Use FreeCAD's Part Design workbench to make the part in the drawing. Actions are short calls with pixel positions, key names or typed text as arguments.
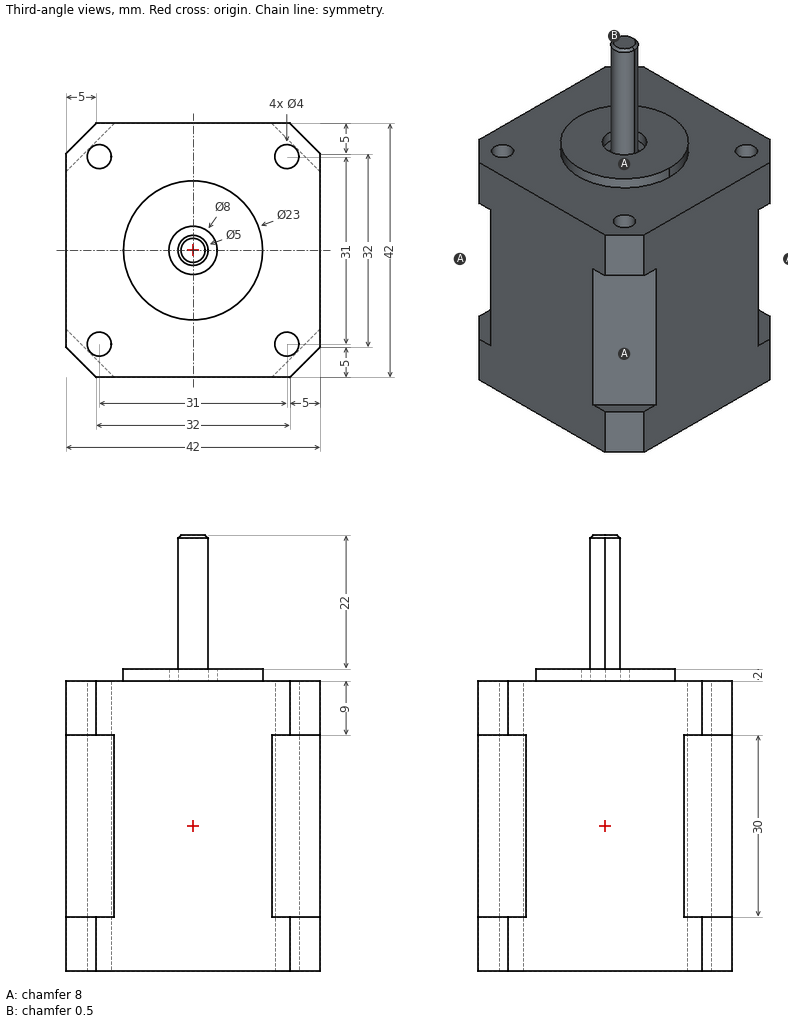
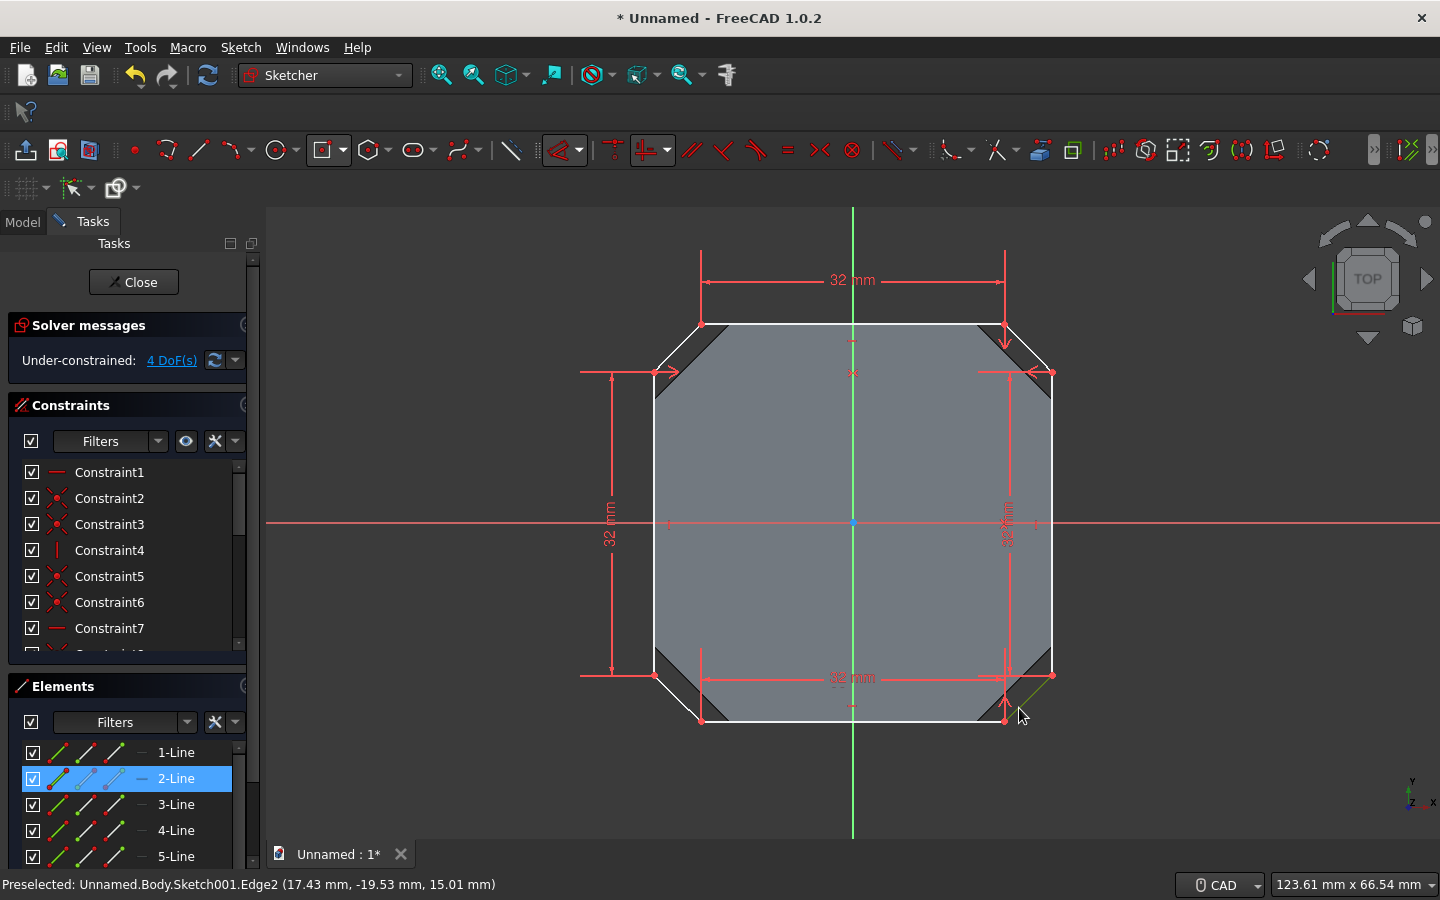
click(582, 150)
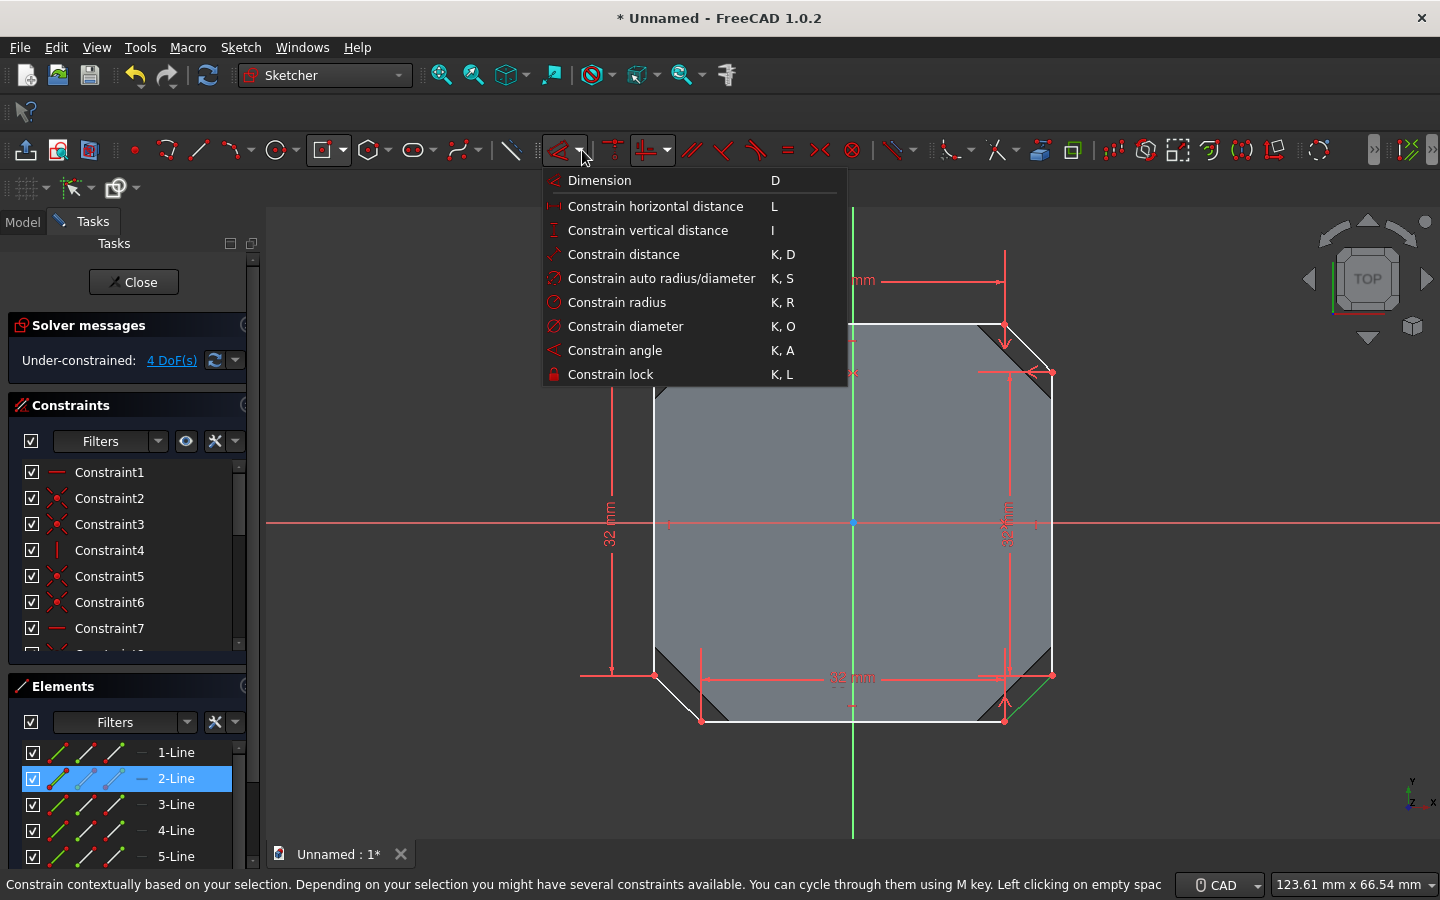
click(695, 206)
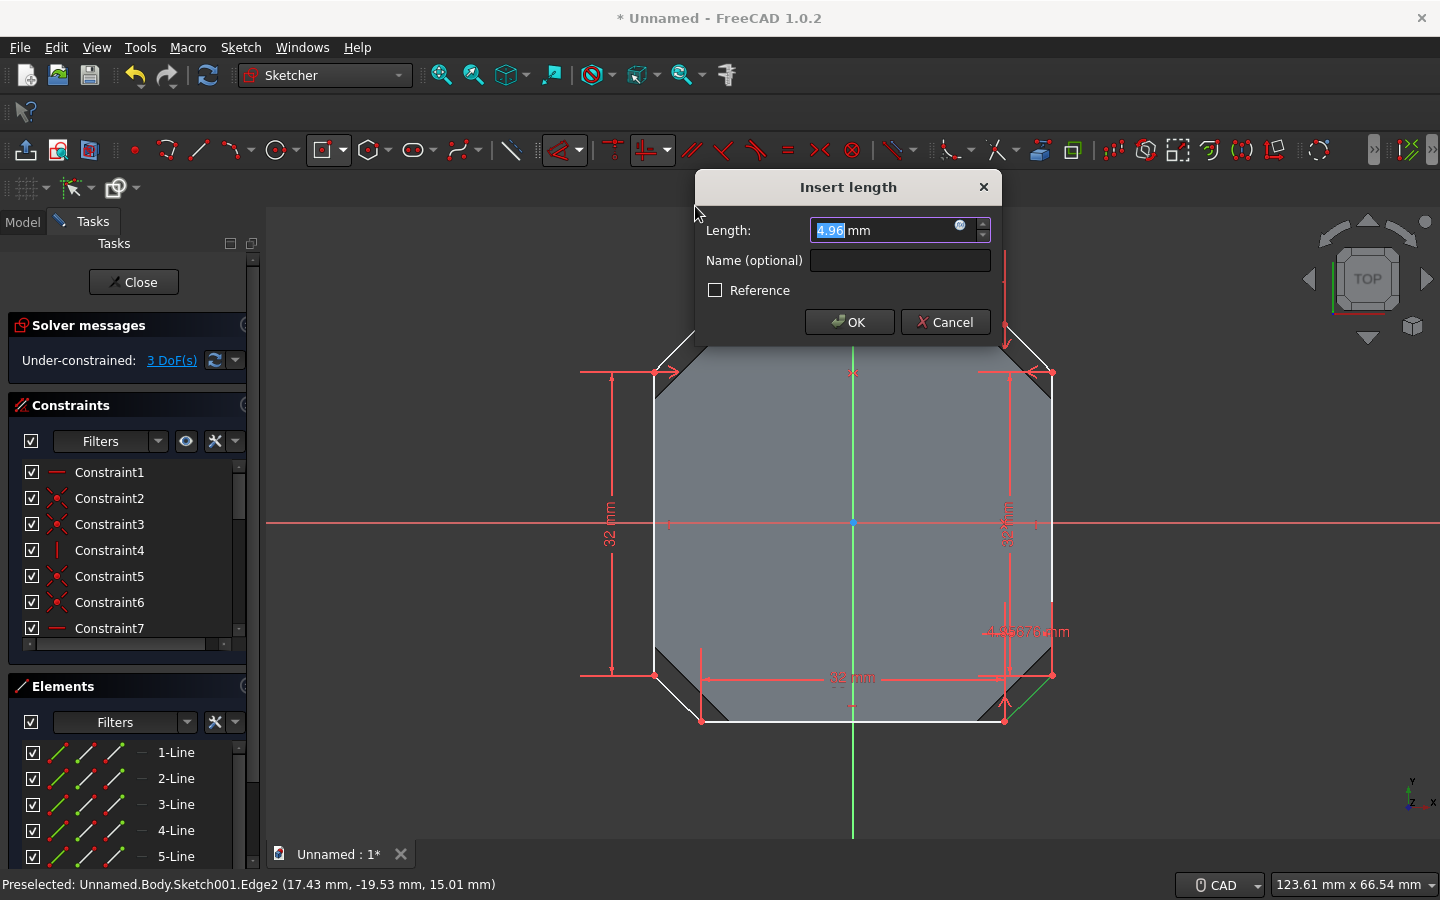
text(5)
key(Return)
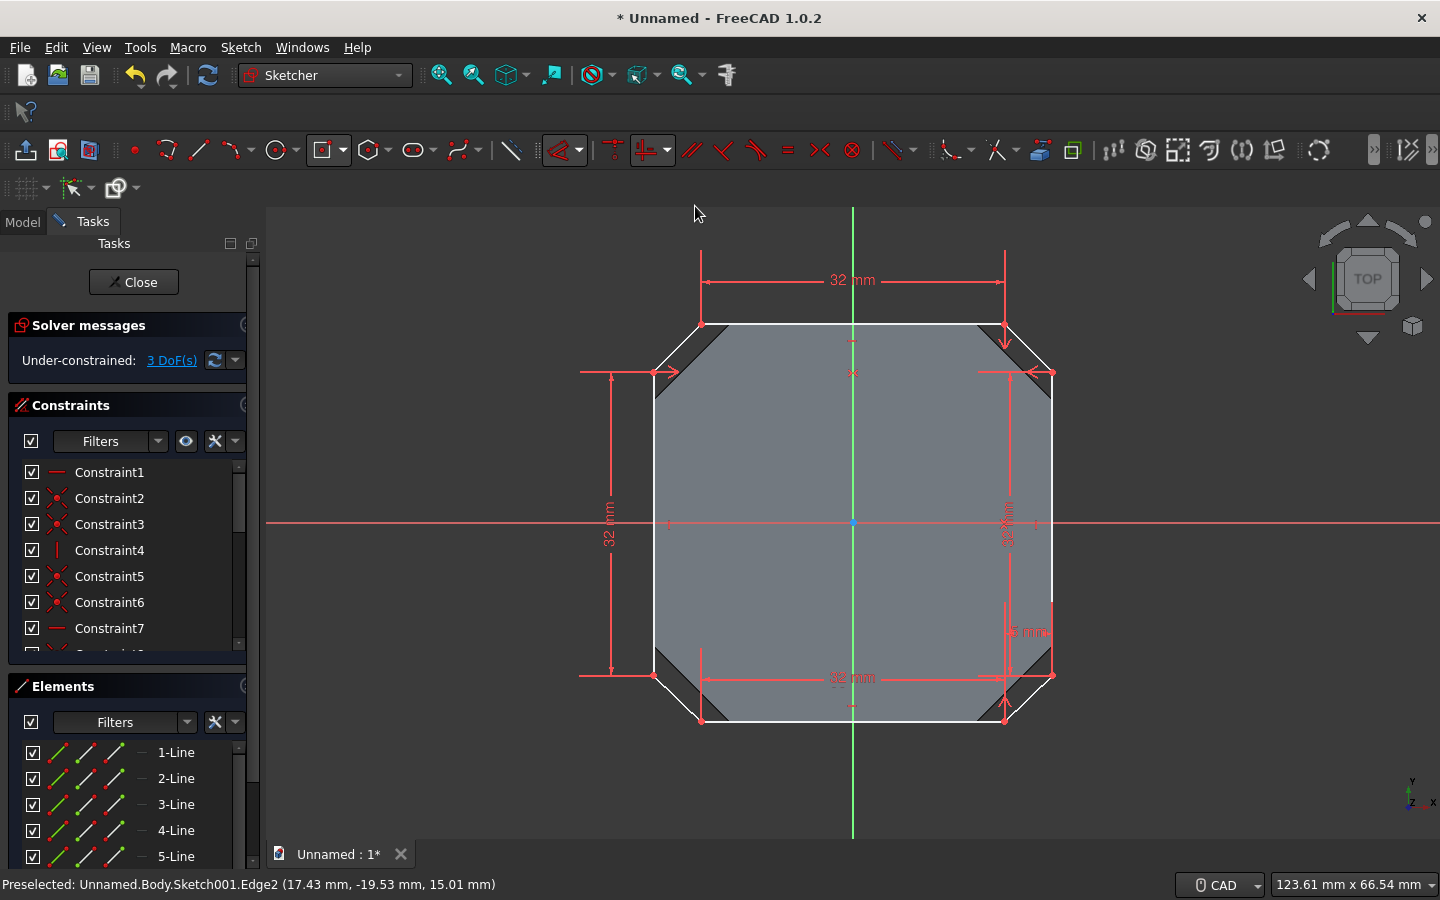
click(1019, 708)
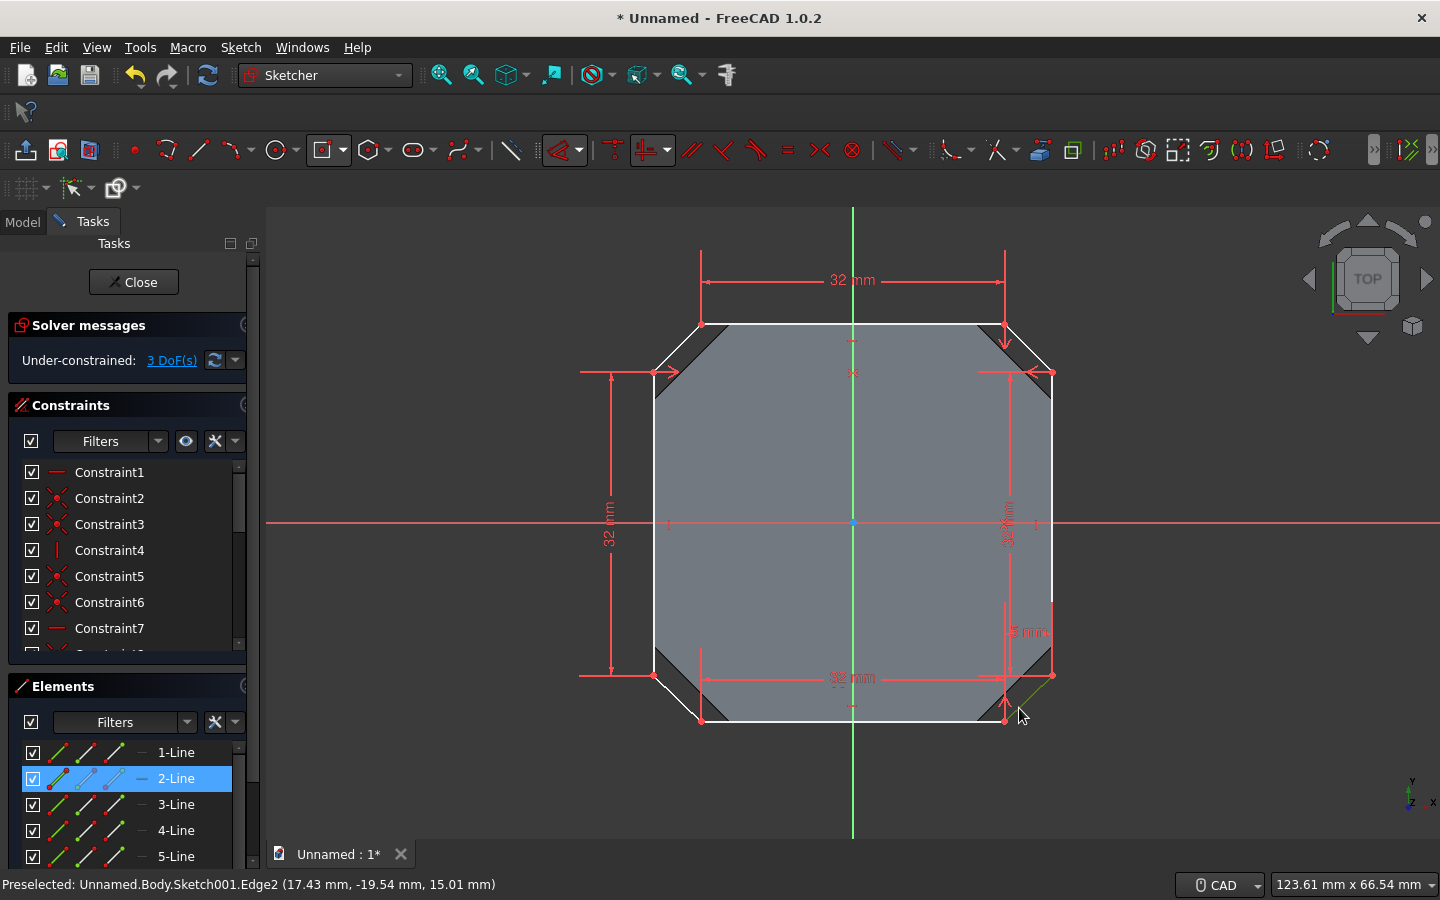
click(582, 150)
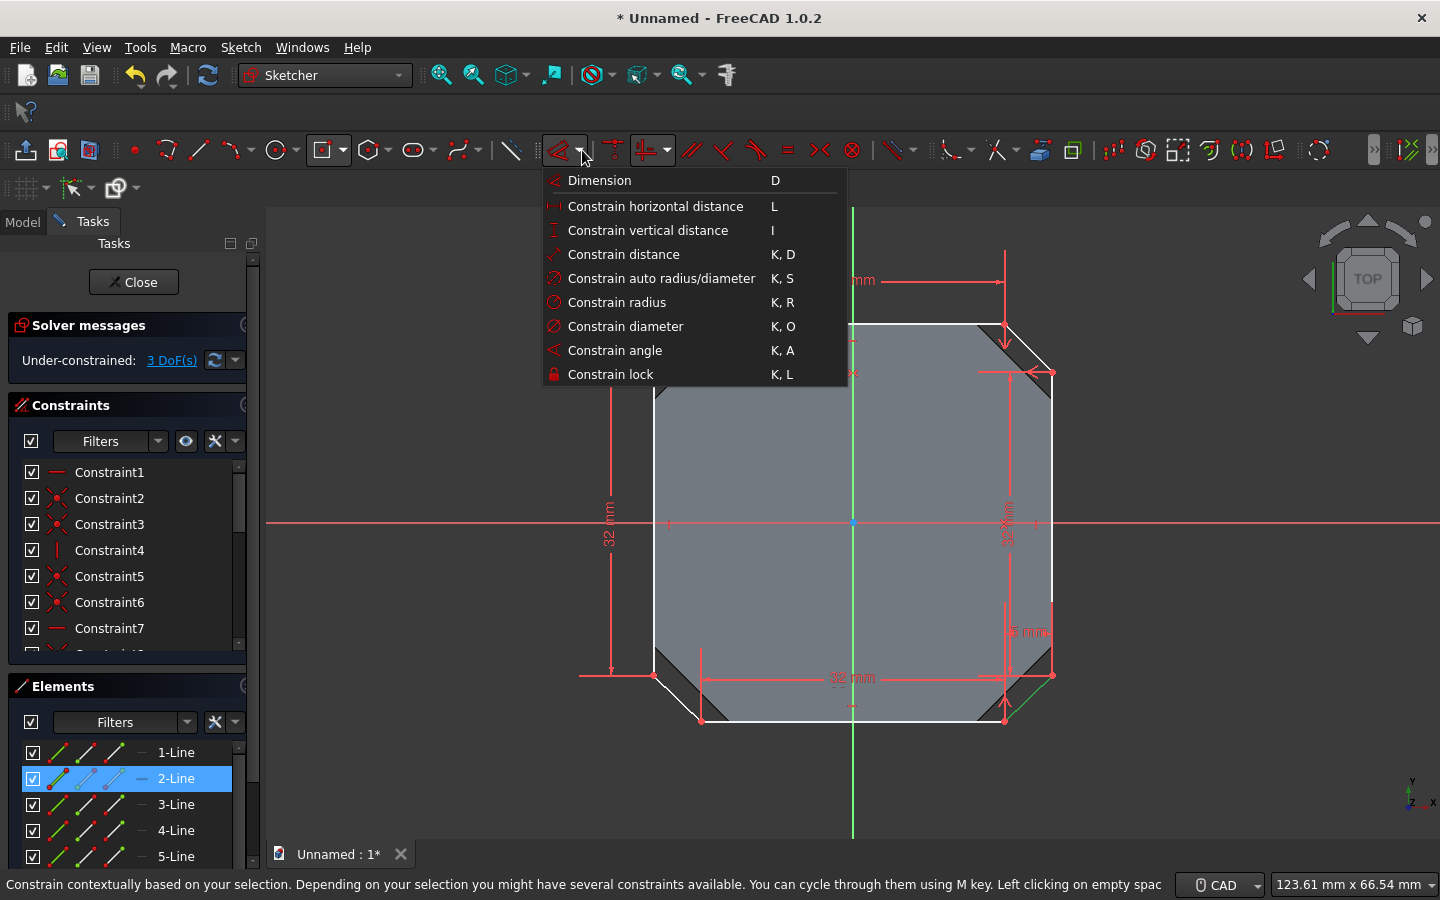
click(695, 230)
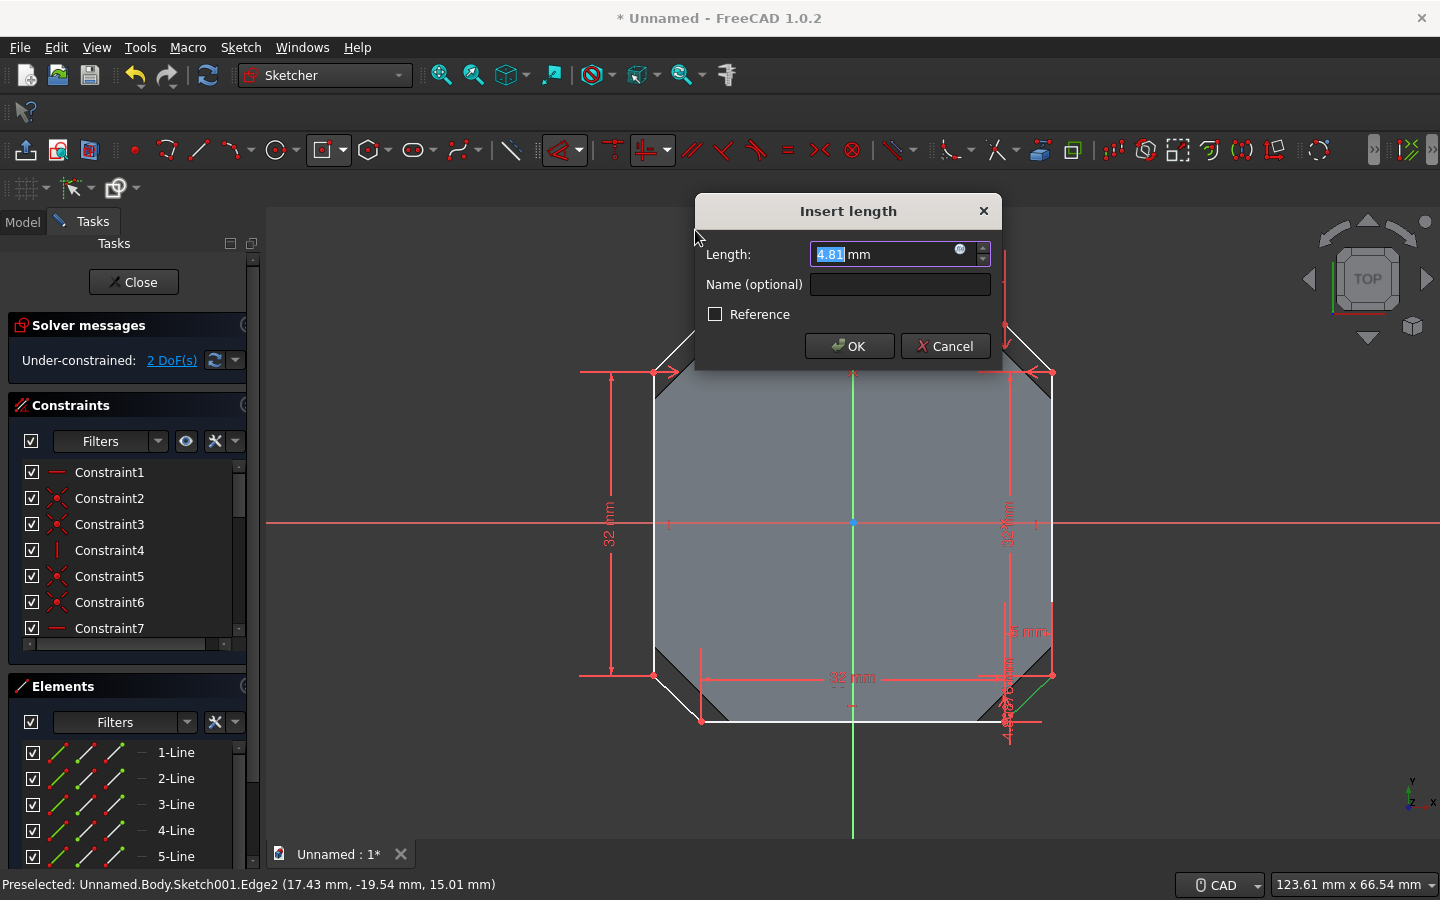
text(5)
key(Return)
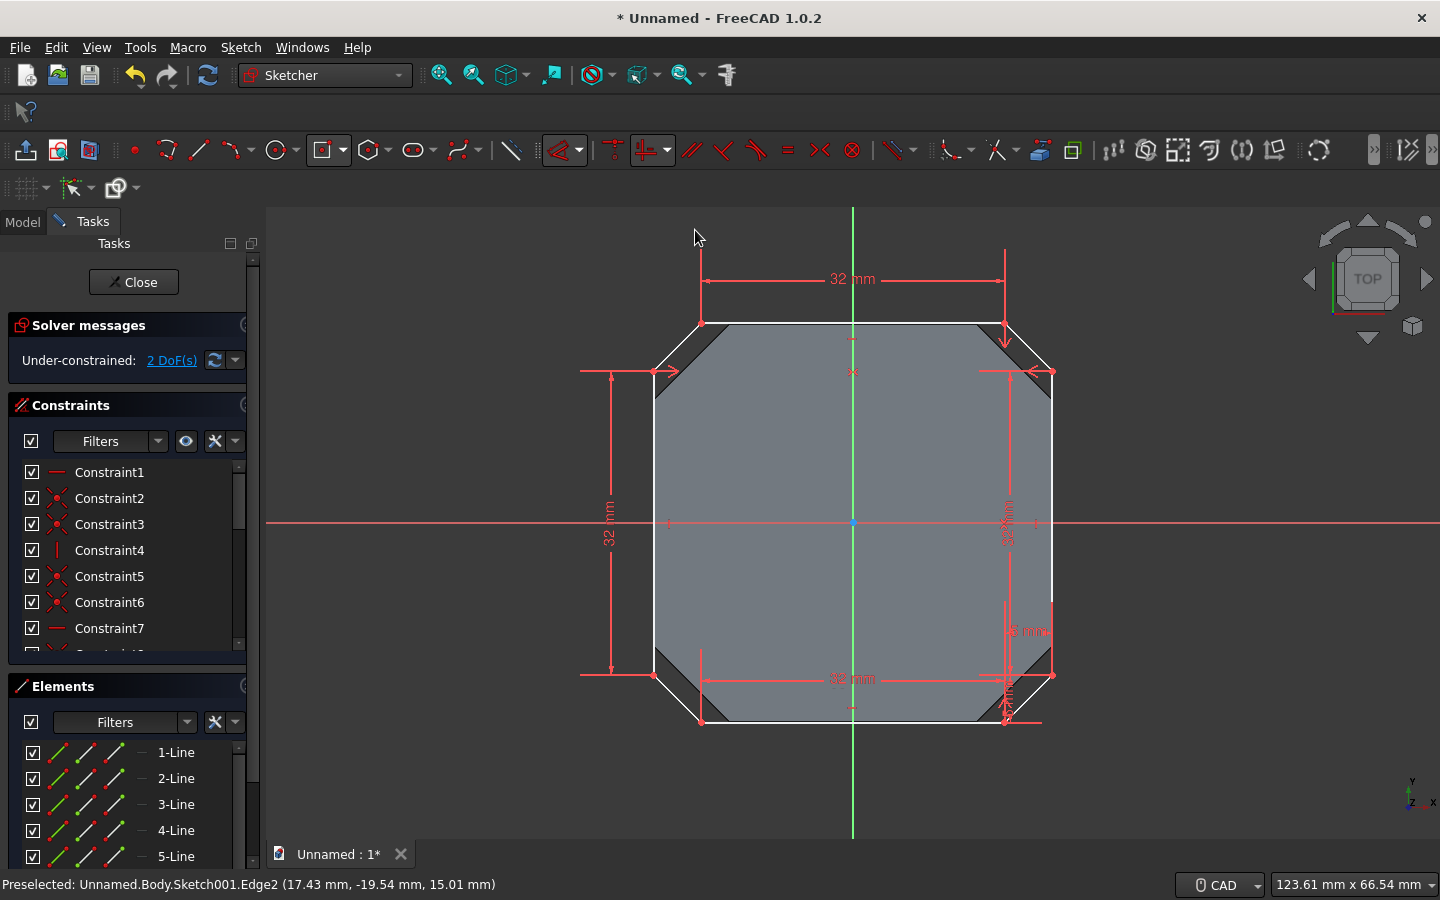
click(1038, 357)